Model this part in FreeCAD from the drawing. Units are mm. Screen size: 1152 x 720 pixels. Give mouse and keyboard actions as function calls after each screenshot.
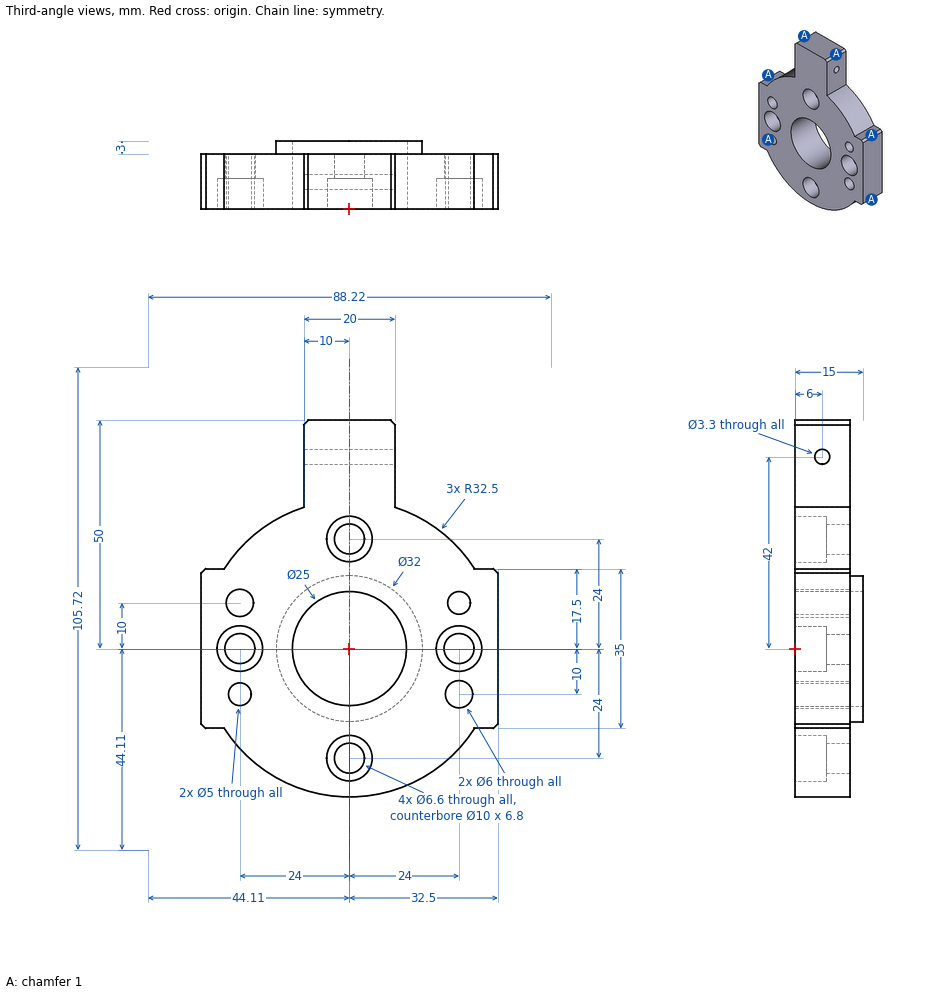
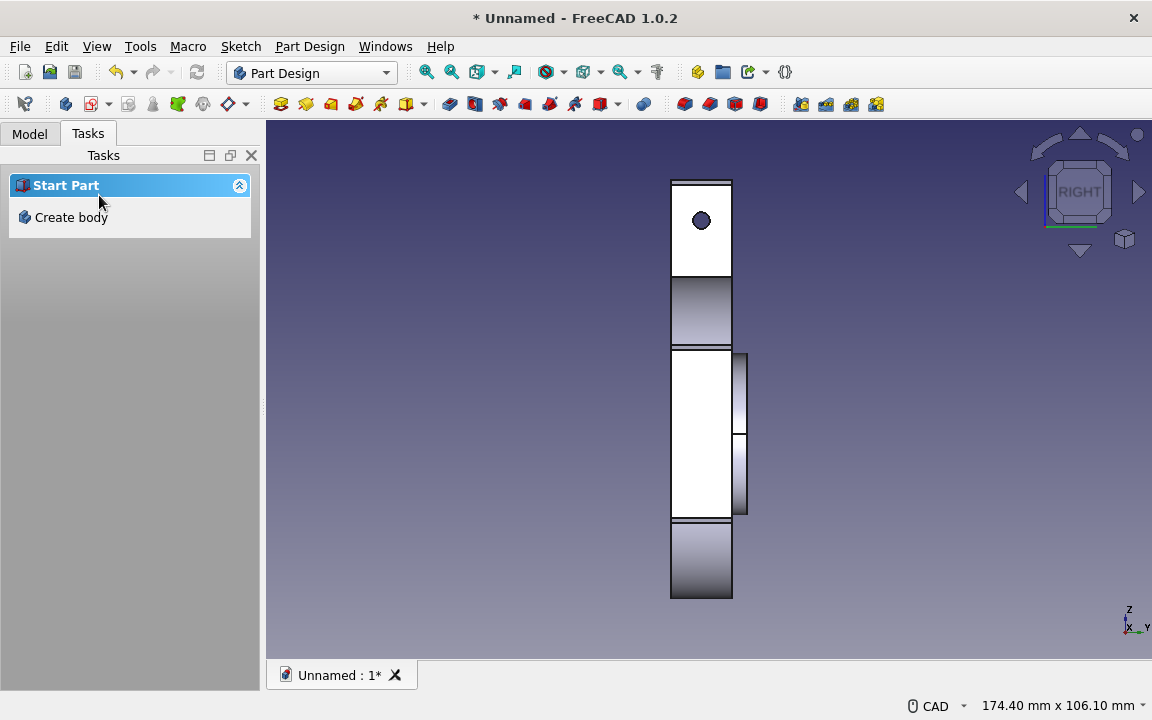
key(0)